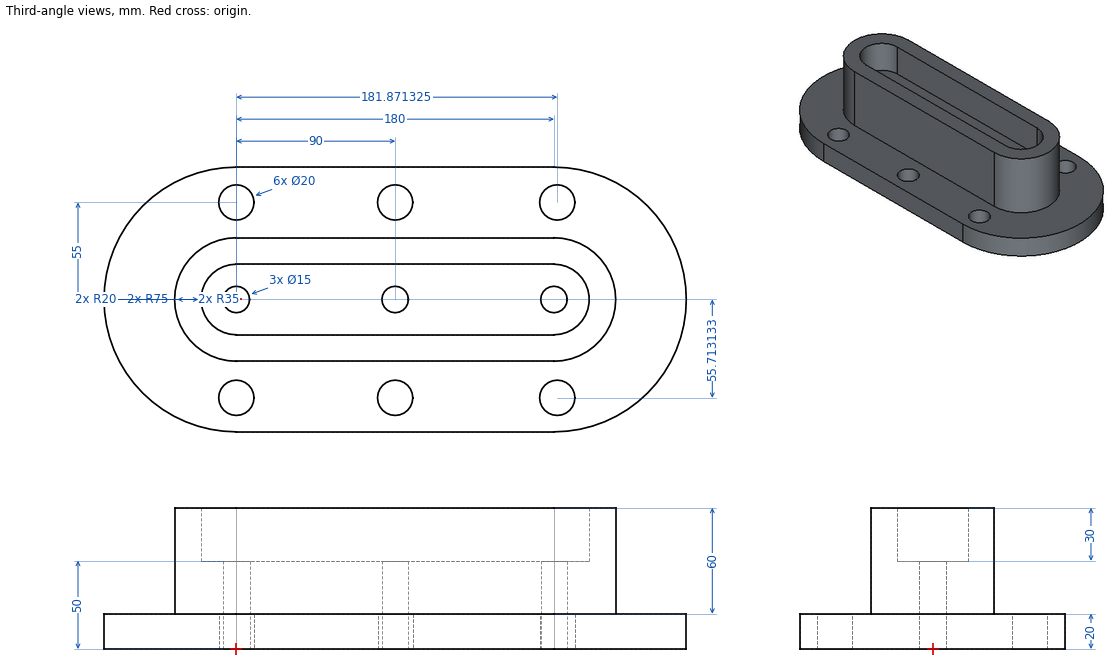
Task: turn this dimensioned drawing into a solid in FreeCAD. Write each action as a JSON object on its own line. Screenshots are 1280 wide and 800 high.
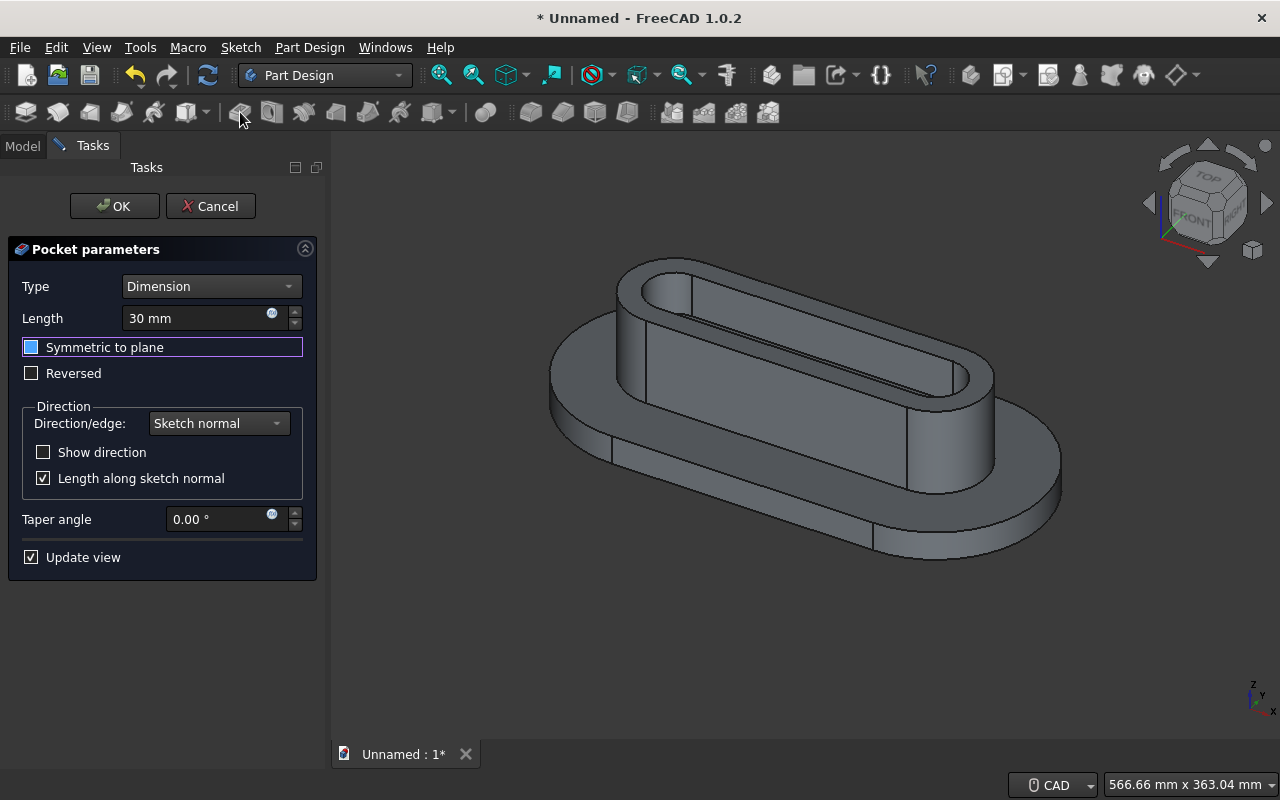
{"action": "left_click", "coordinate": [115, 206]}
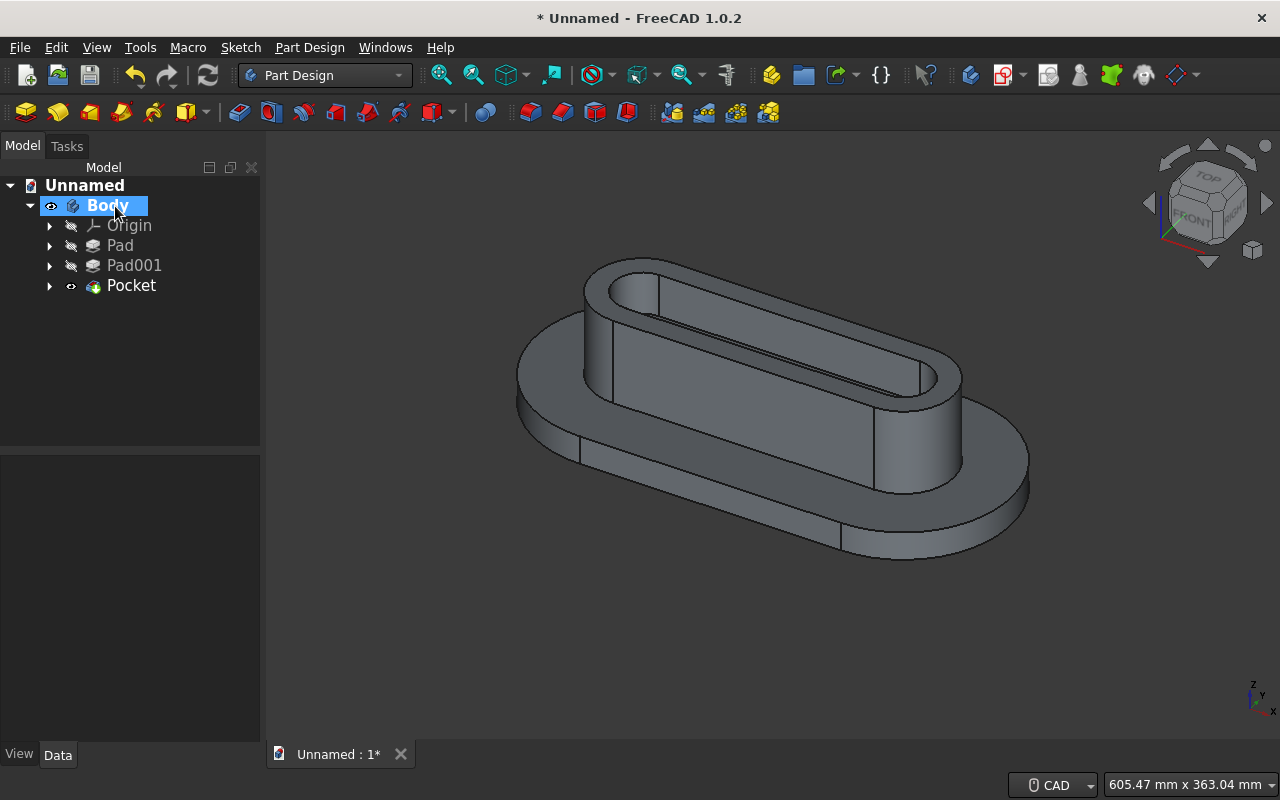
{"action": "key", "text": "0"}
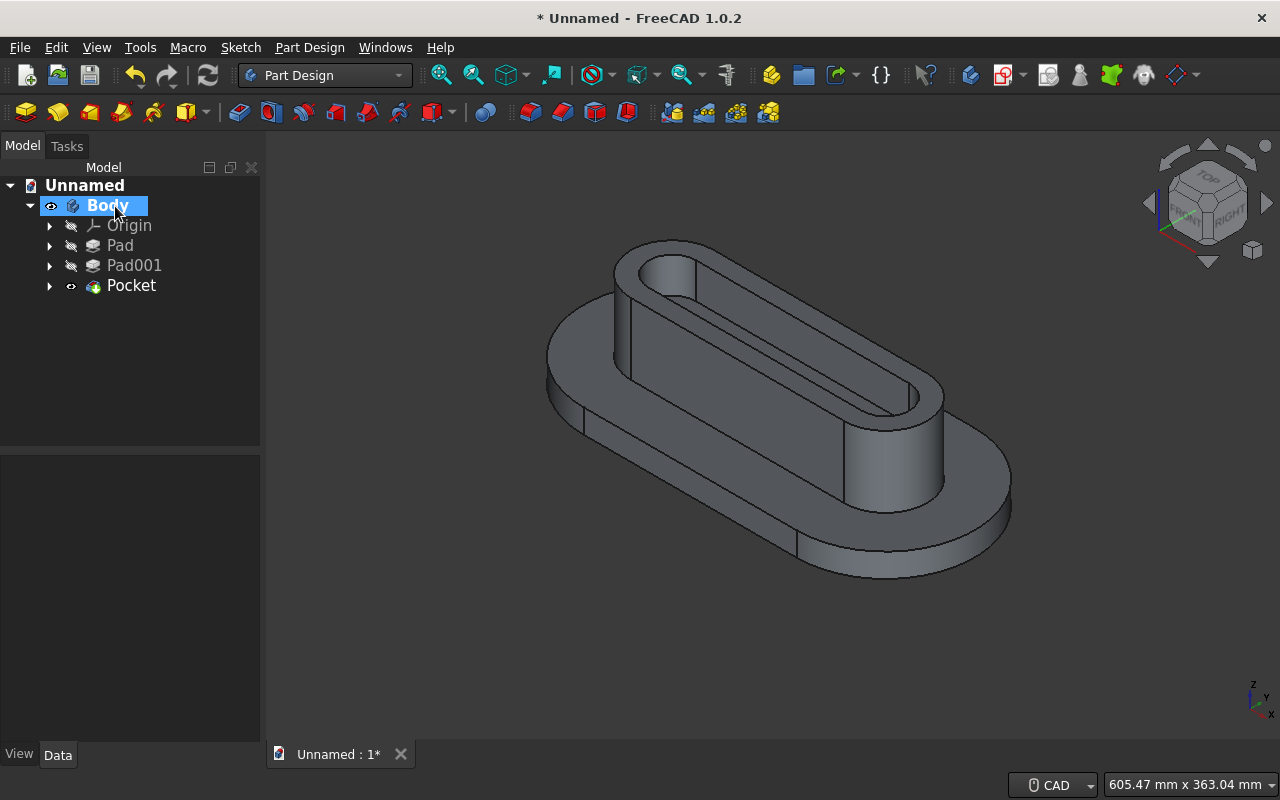
{"action": "key", "text": "2"}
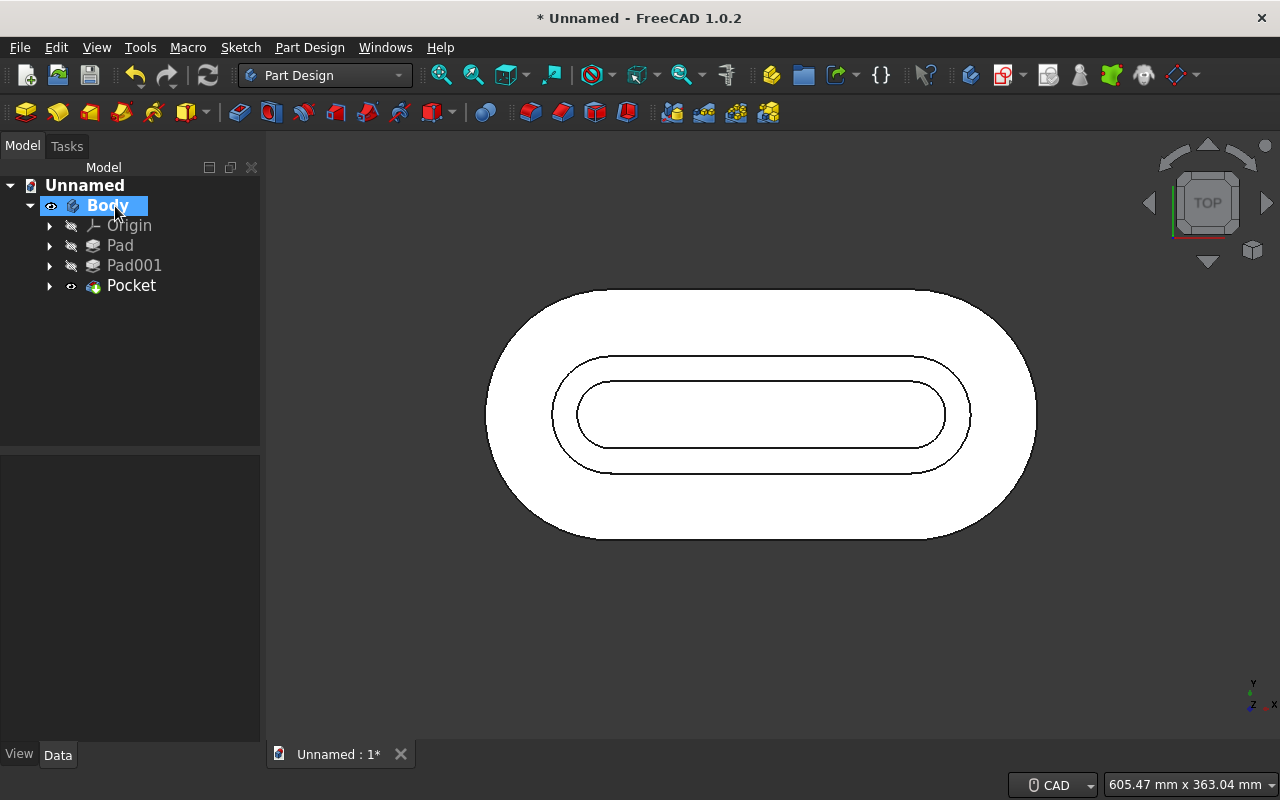
{"action": "left_click", "coordinate": [867, 414]}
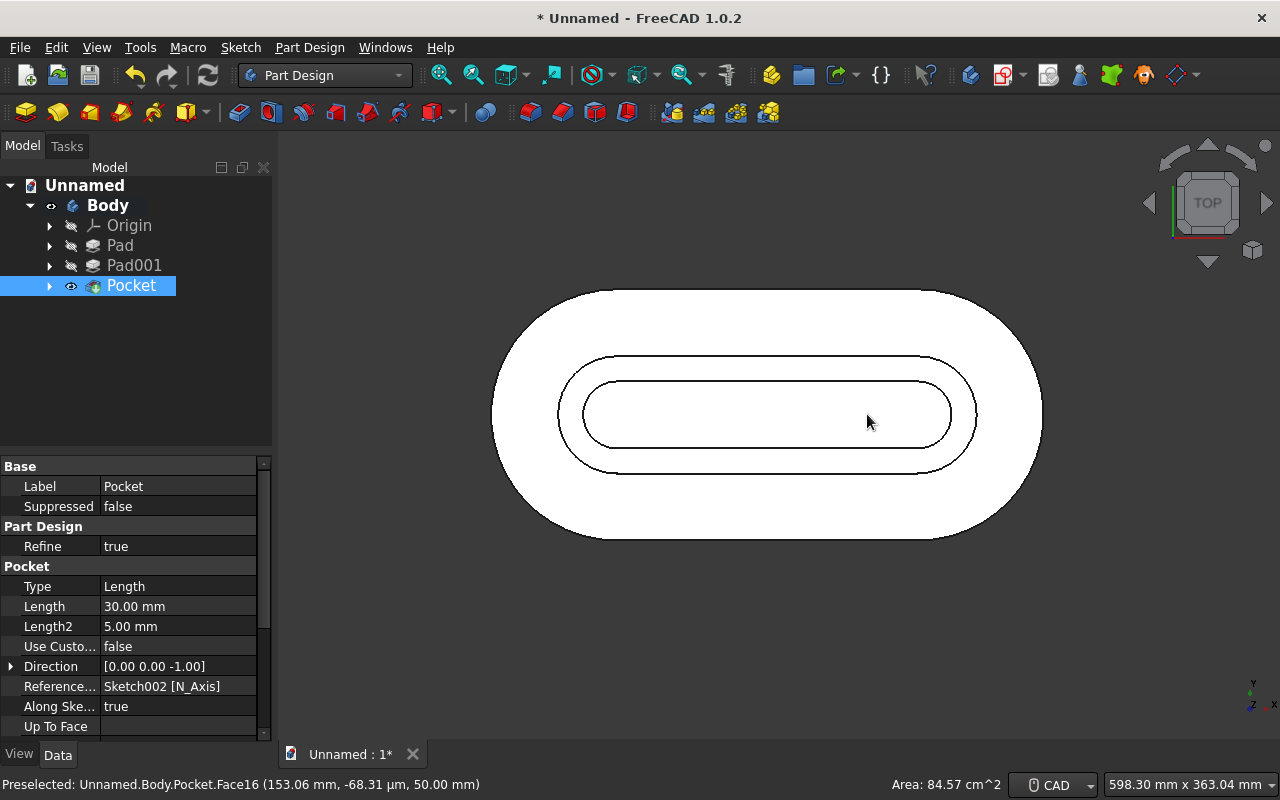
{"action": "left_click", "coordinate": [1004, 76]}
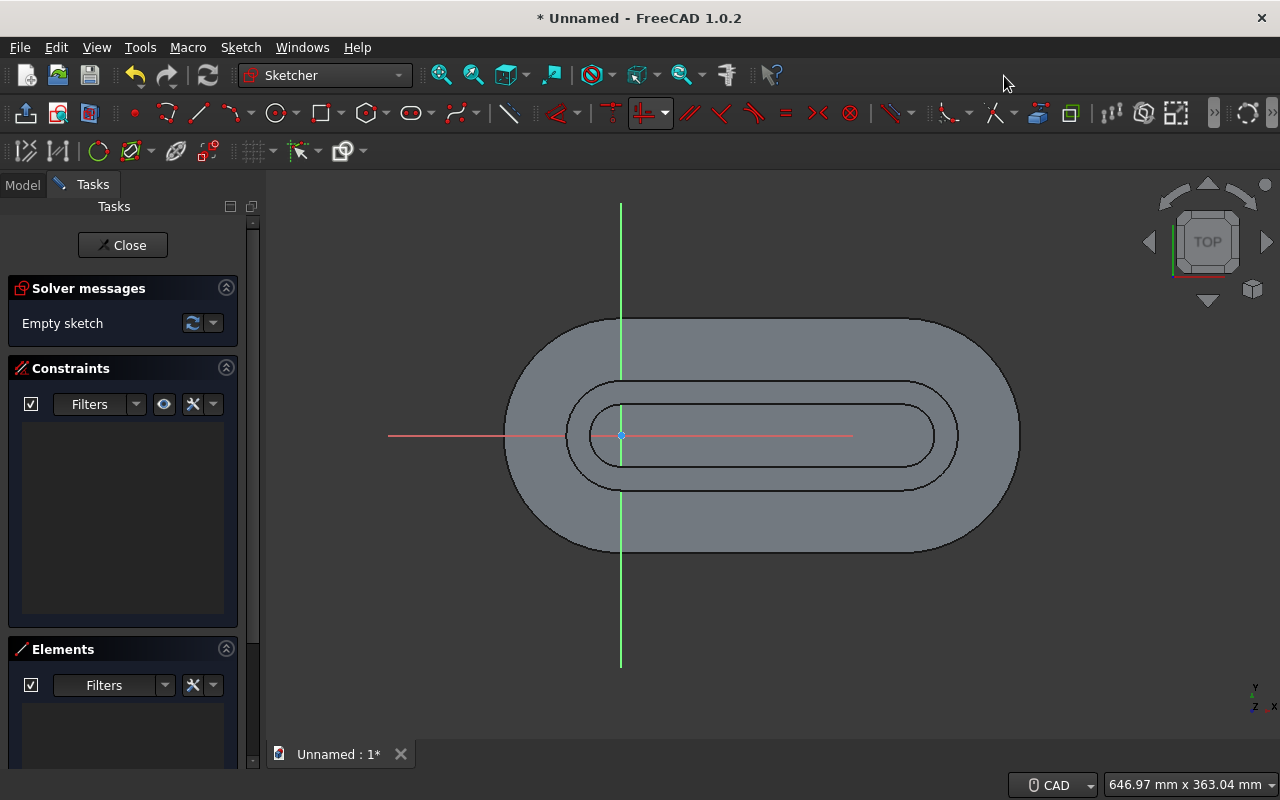
{"action": "scroll", "coordinate": [832, 413], "scroll_direction": "up", "scroll_amount": 3}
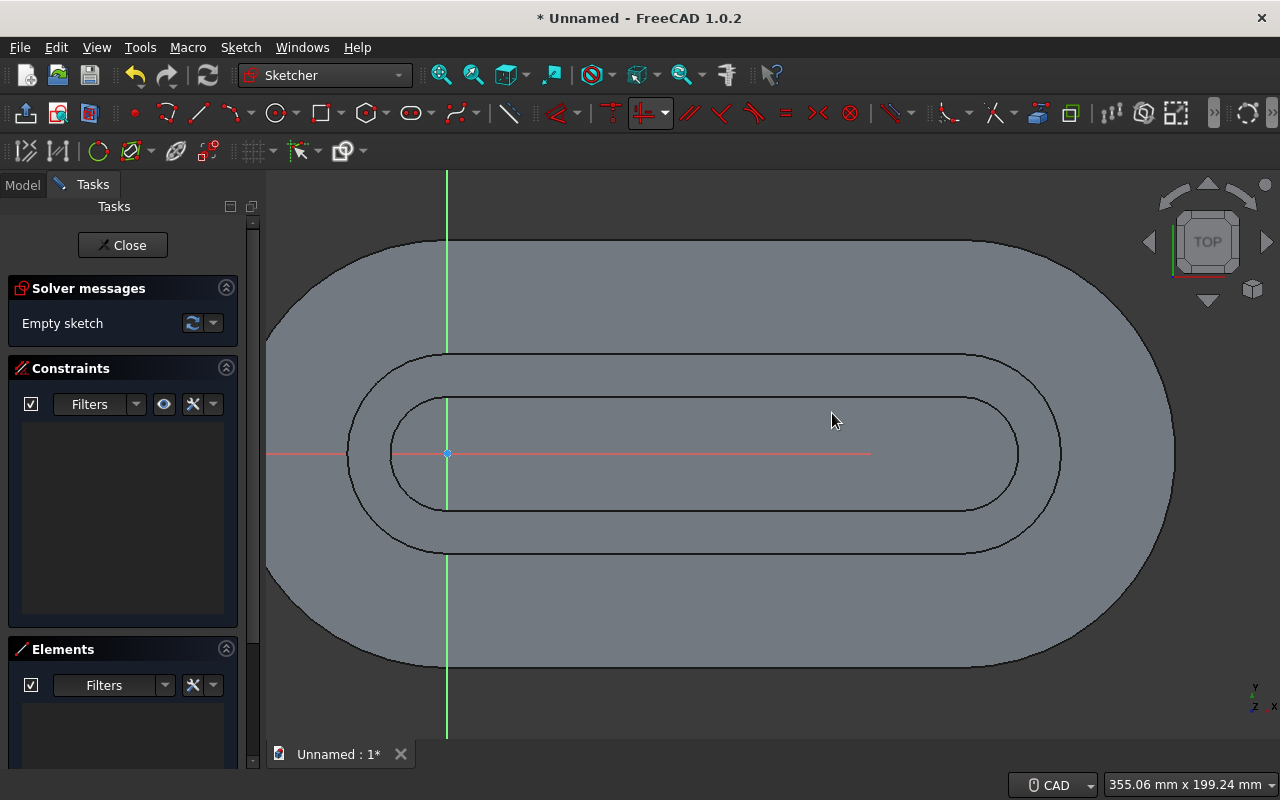
{"action": "left_click", "coordinate": [276, 114]}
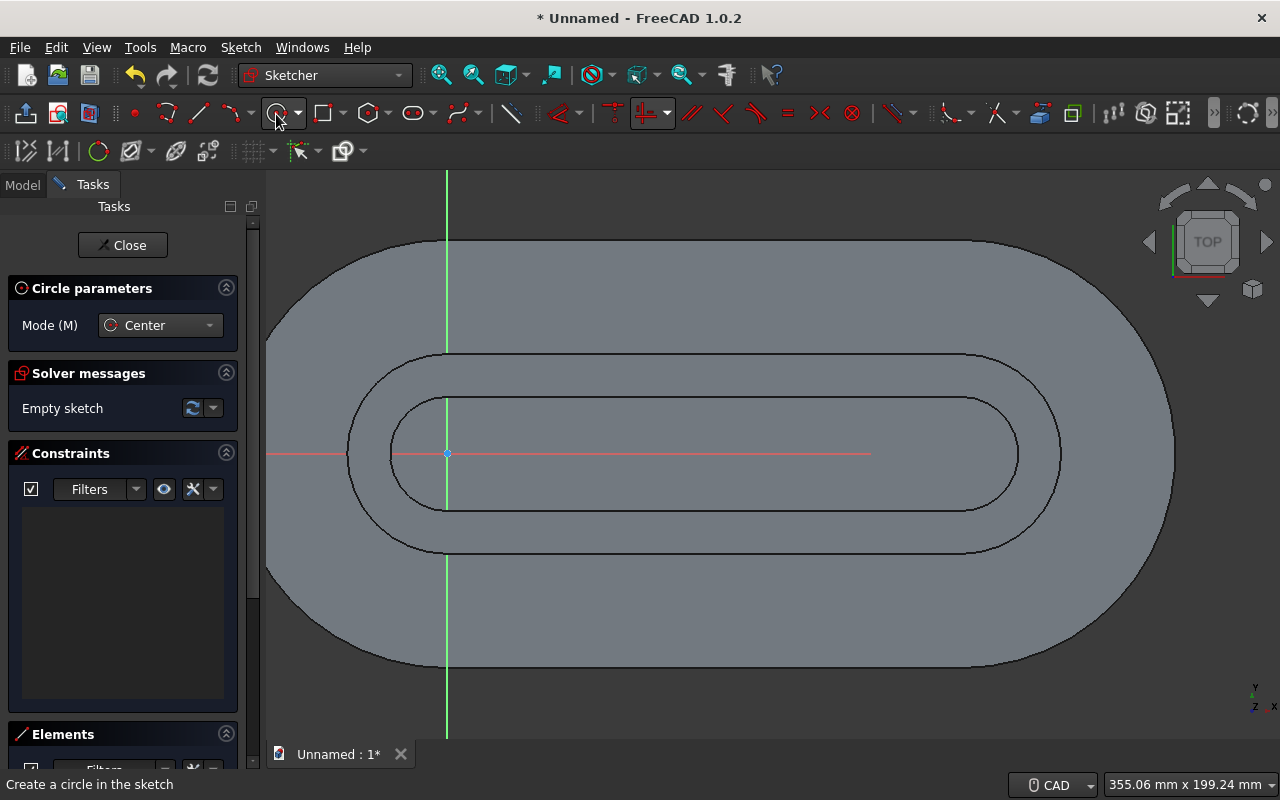
{"action": "left_click", "coordinate": [447, 454]}
{"action": "mouse_move", "coordinate": [462, 439]}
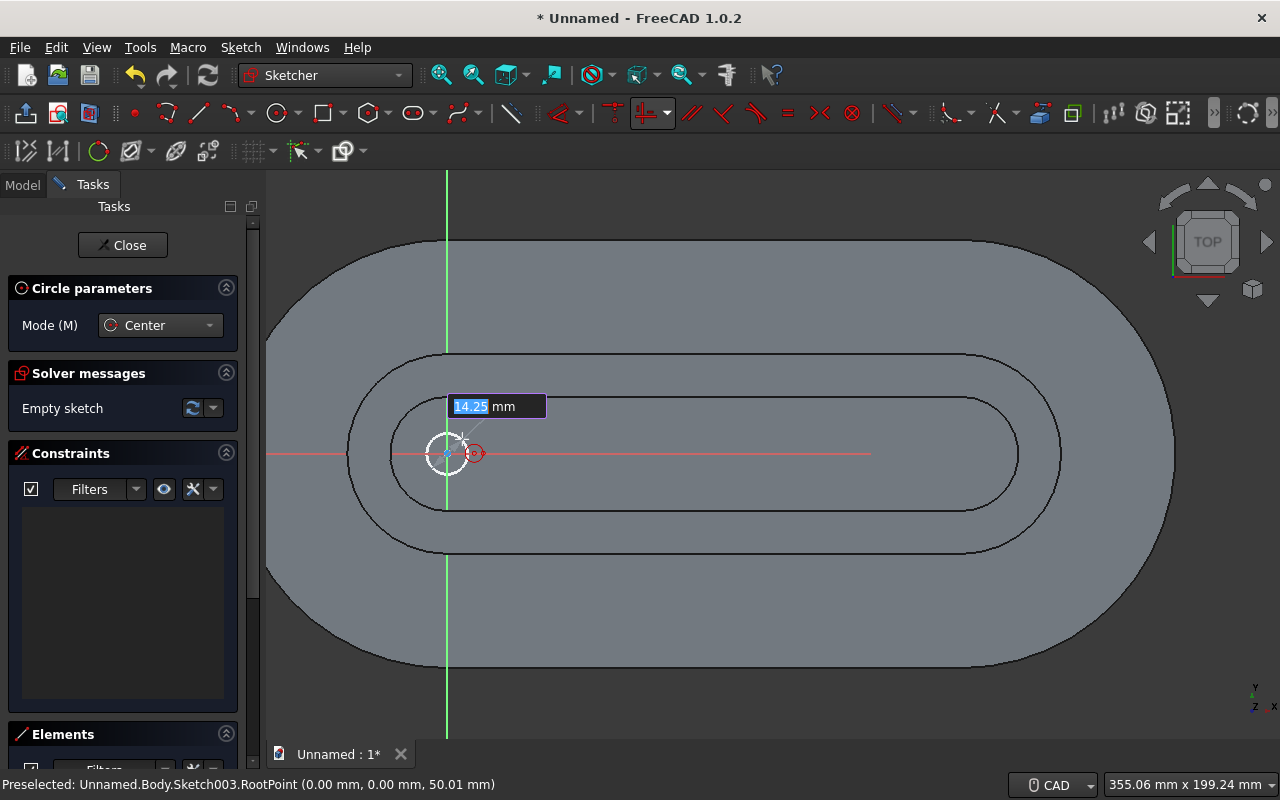
{"action": "type", "text": "15"}
{"action": "key", "text": "Return"}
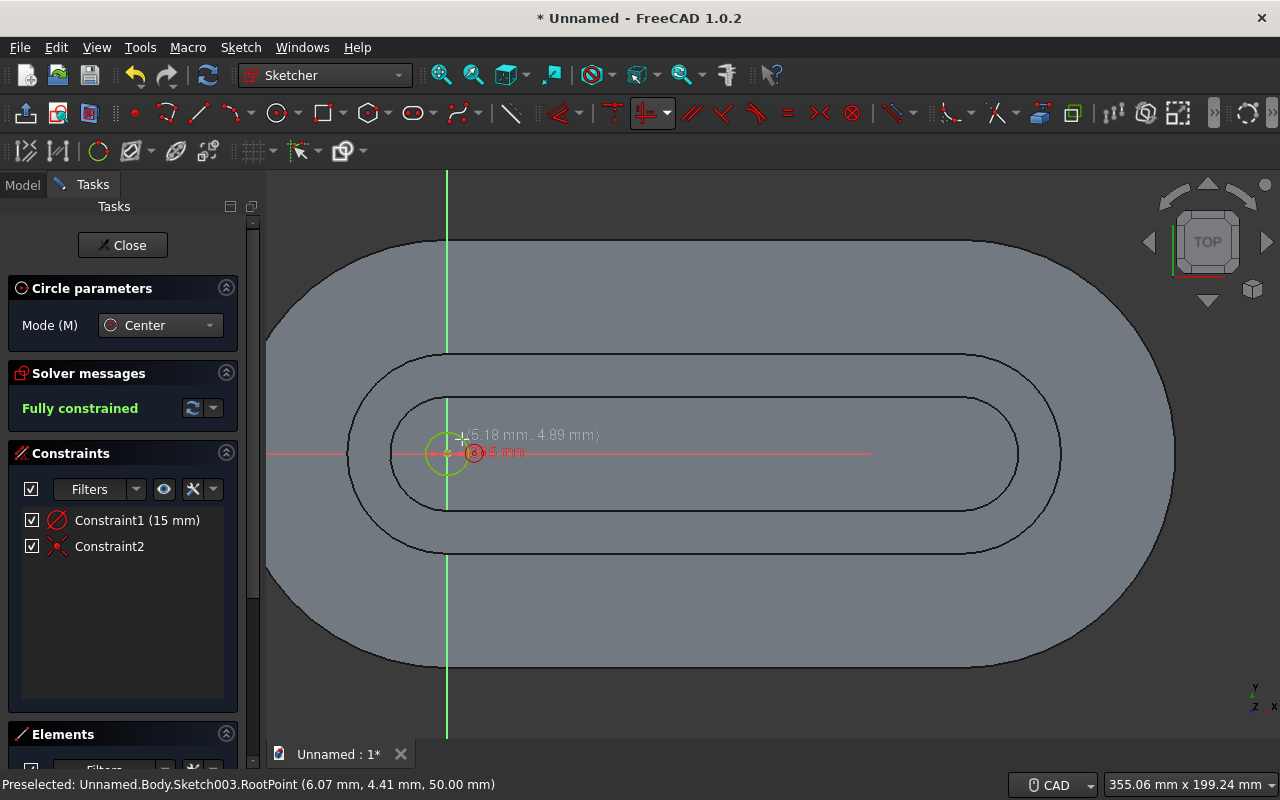
{"action": "left_click", "coordinate": [961, 454]}
{"action": "mouse_move", "coordinate": [976, 439]}